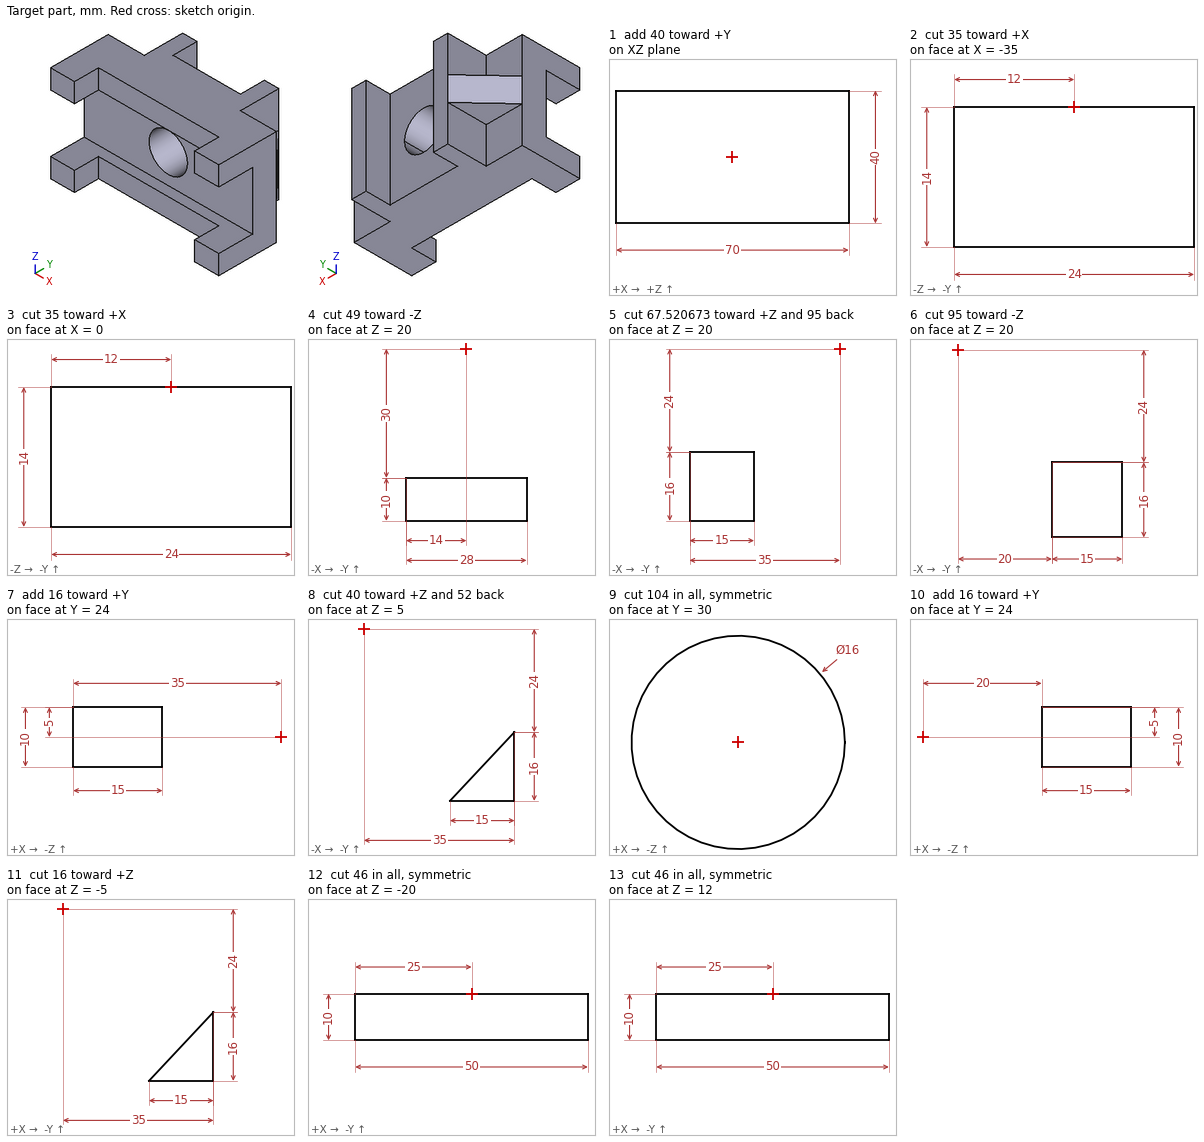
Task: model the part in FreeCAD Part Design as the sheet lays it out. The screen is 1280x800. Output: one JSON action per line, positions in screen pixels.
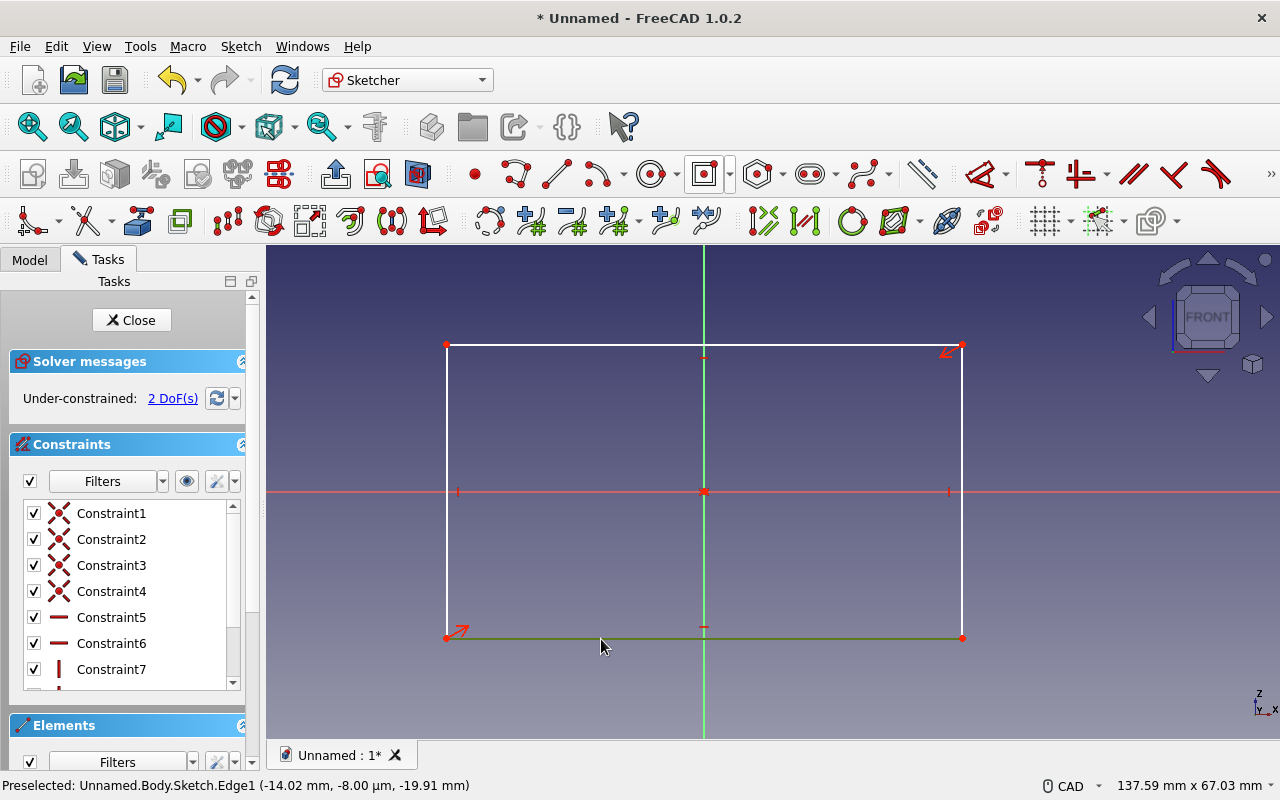
{"action": "key", "text": "l"}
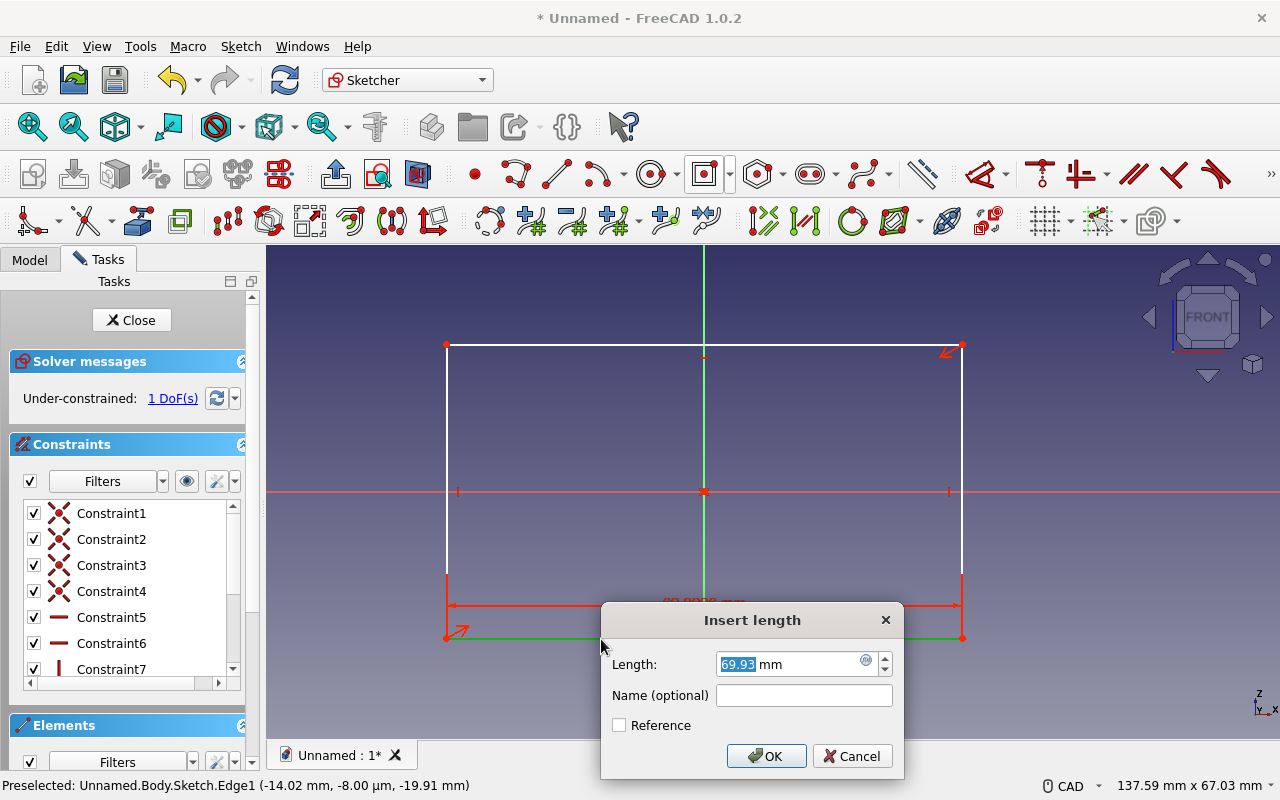
{"action": "type", "text": "70"}
{"action": "key", "text": "Return"}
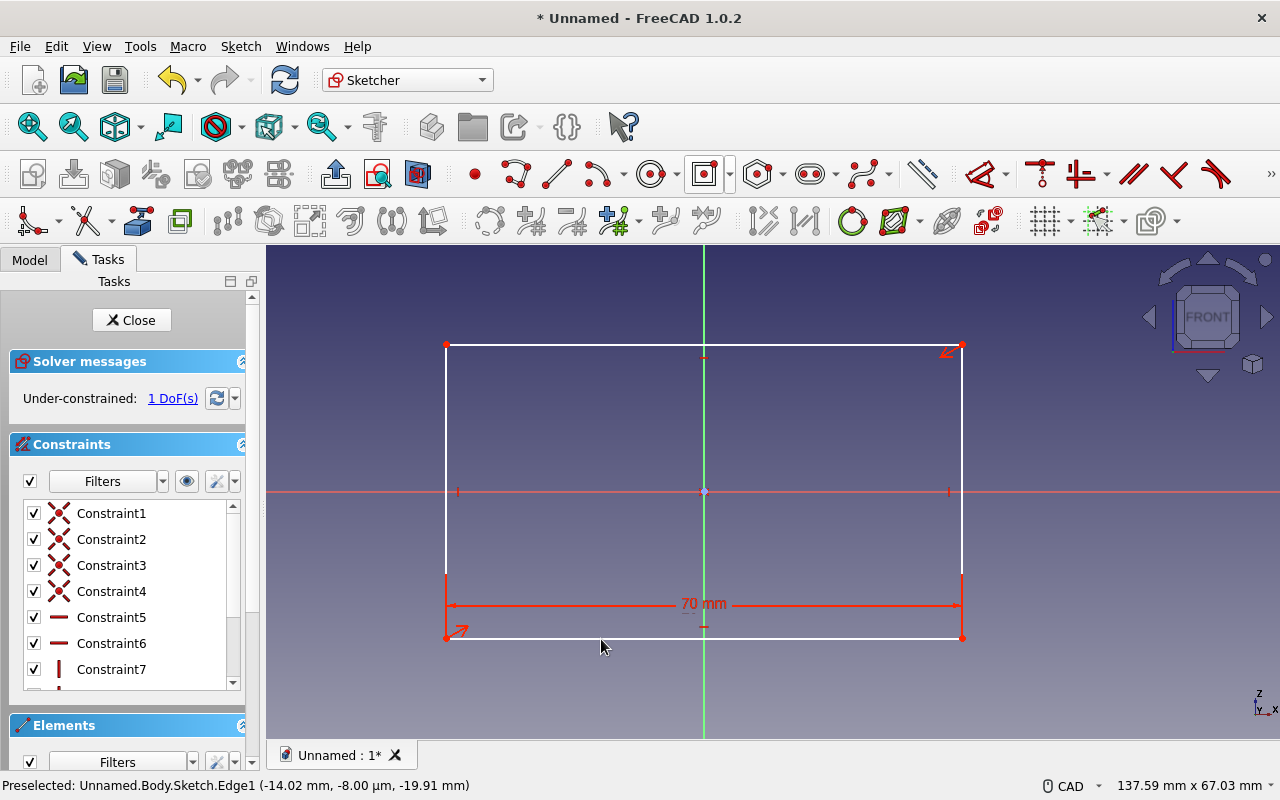
{"action": "left_click", "coordinate": [962, 550]}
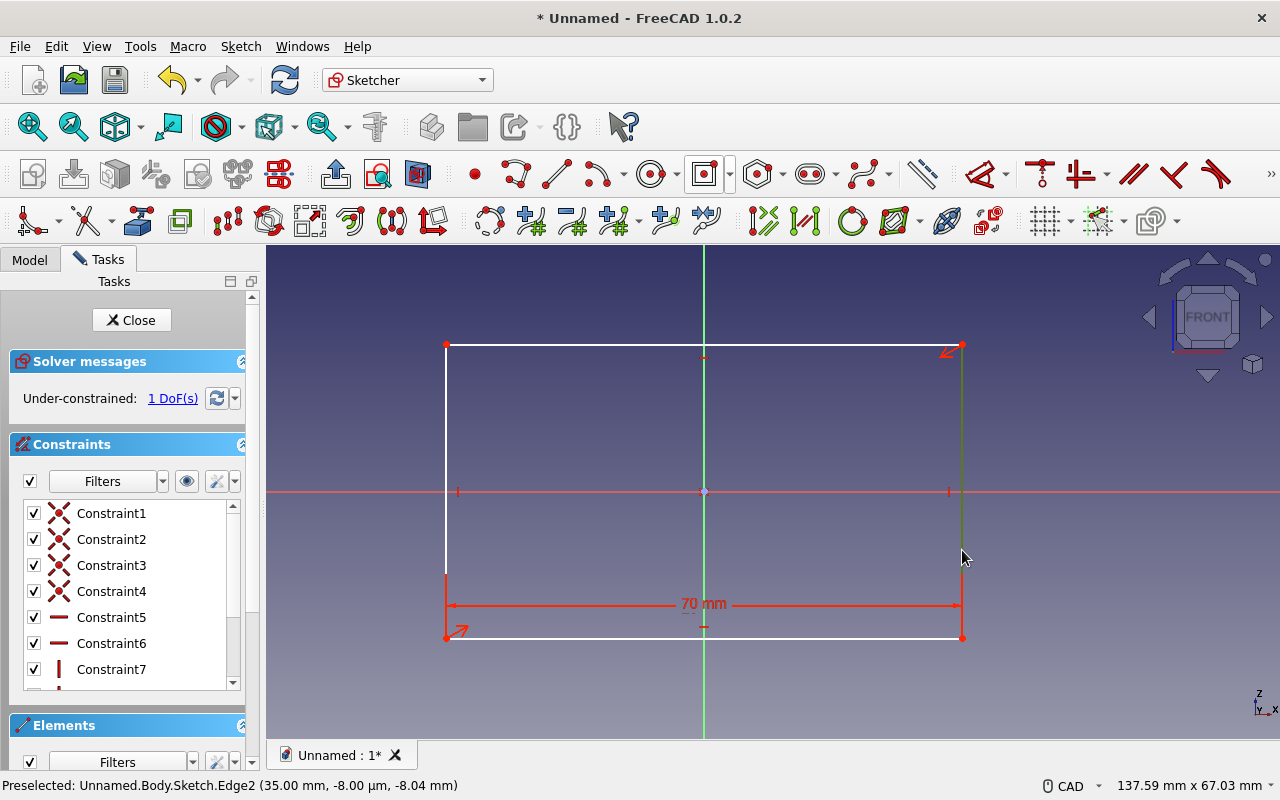
{"action": "key", "text": "i"}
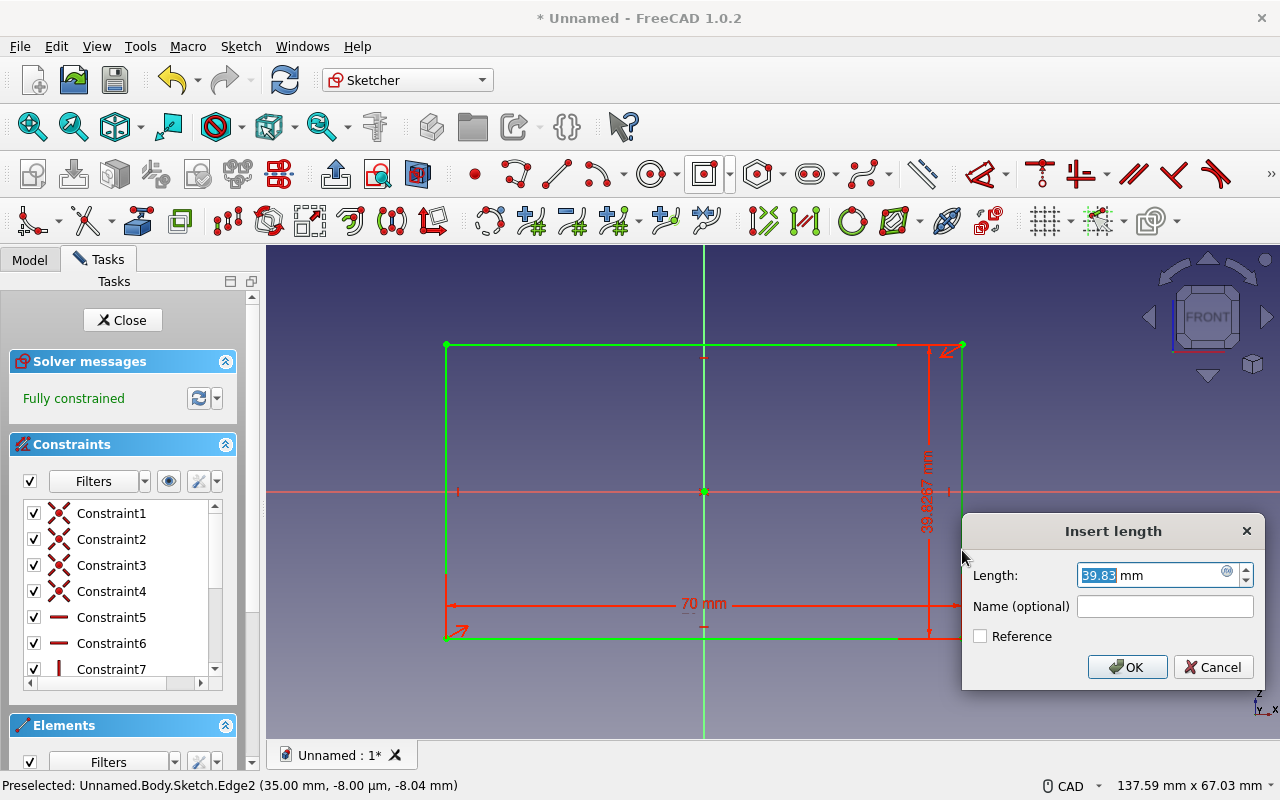
{"action": "type", "text": "40"}
{"action": "key", "text": "Return"}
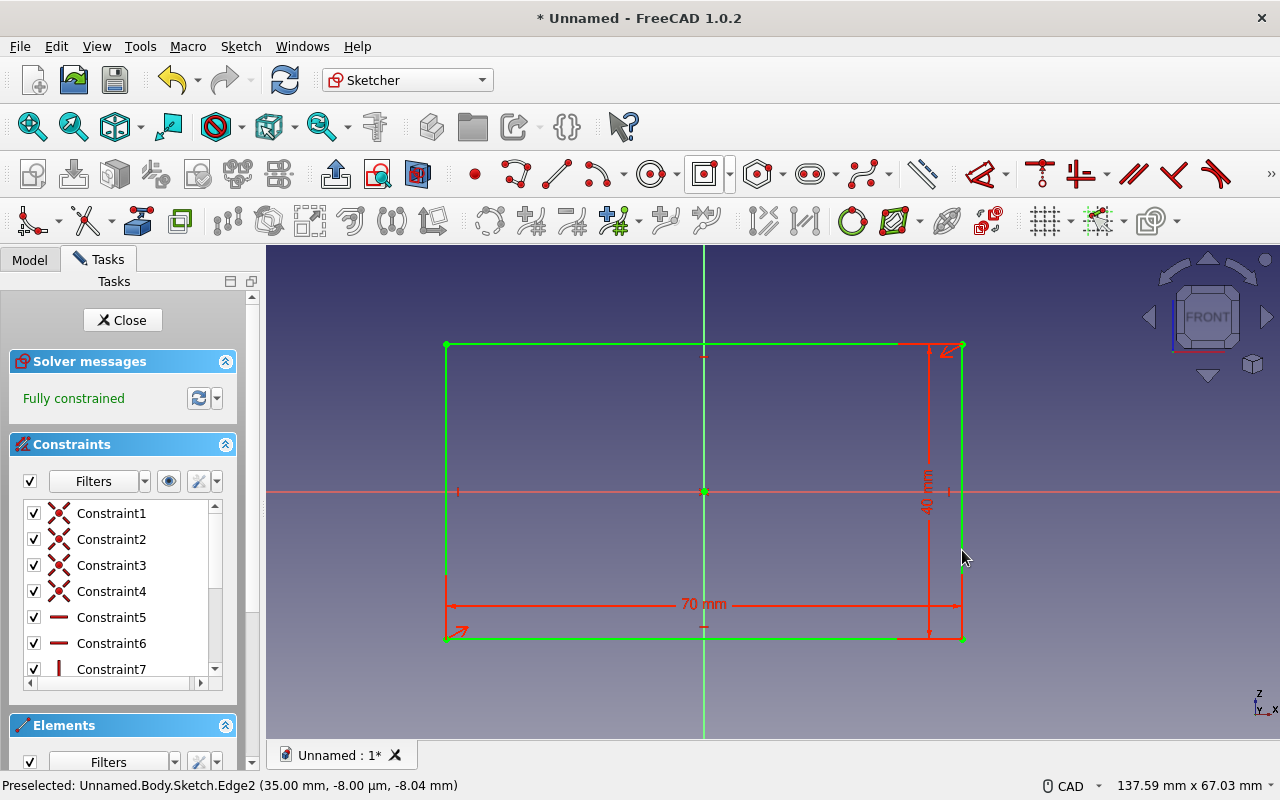
{"action": "left_click", "coordinate": [123, 320]}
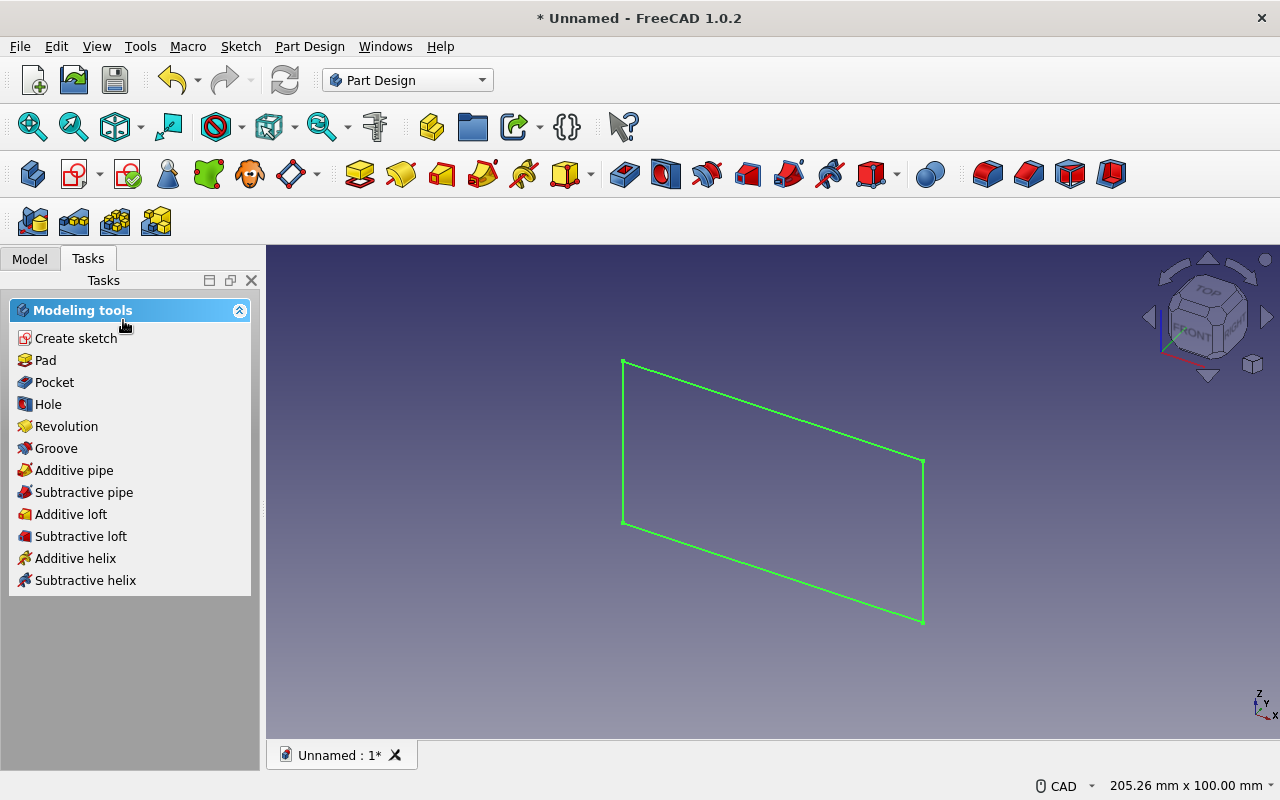
{"action": "left_click", "coordinate": [360, 174]}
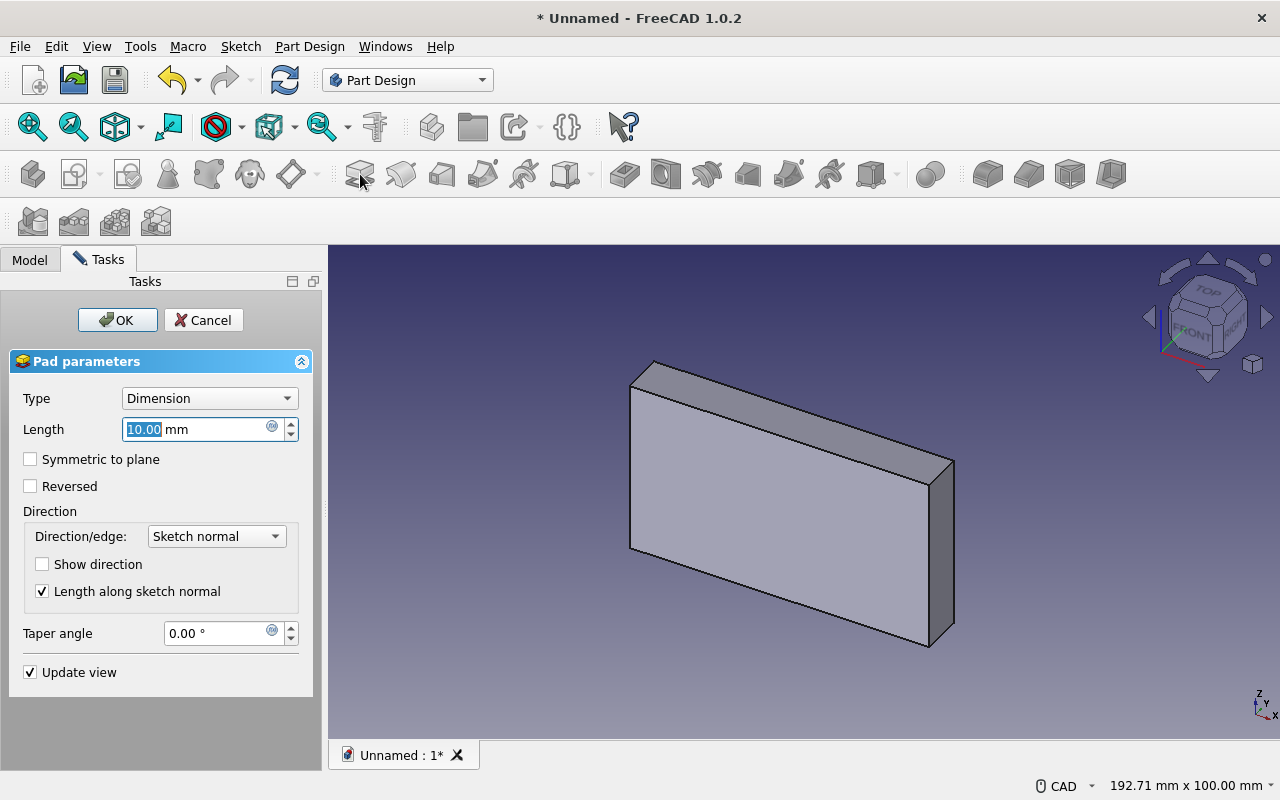
{"action": "type", "text": "40"}
{"action": "key", "text": "Tab"}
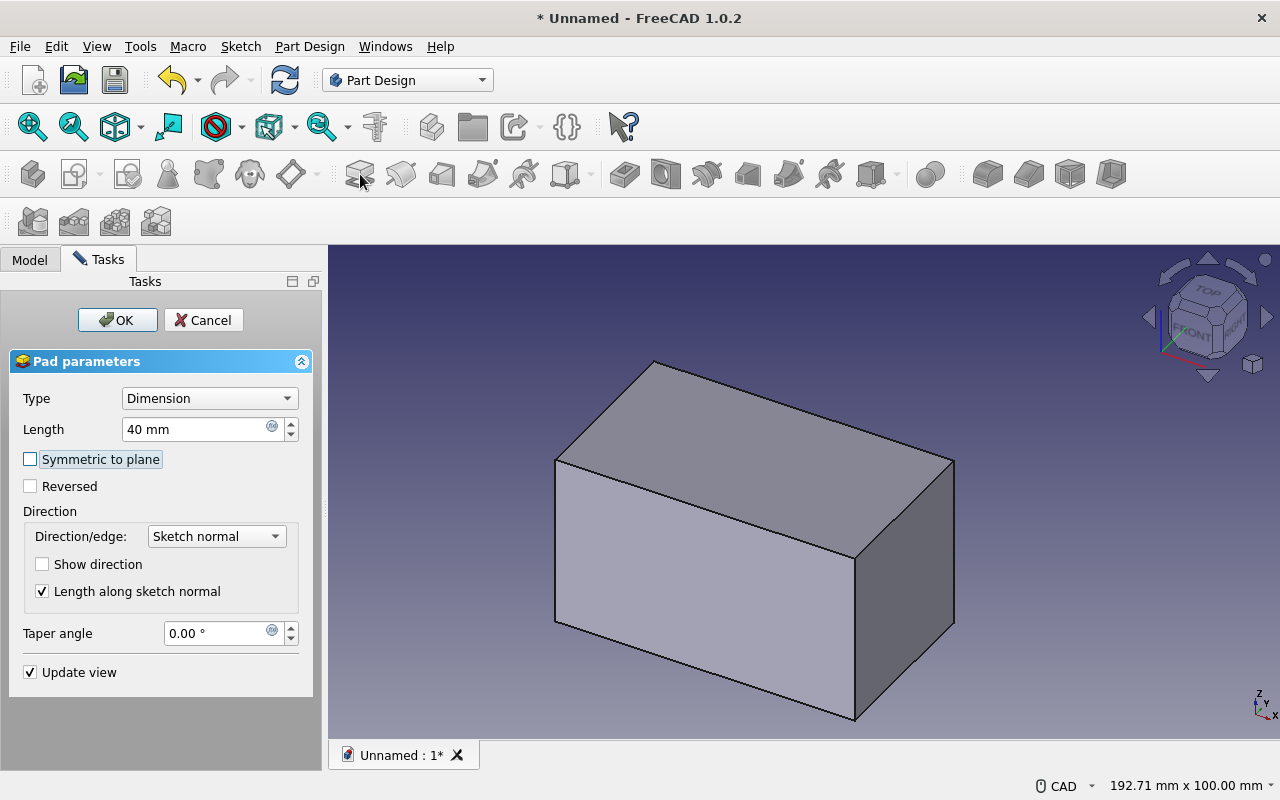
{"action": "left_click", "coordinate": [31, 486]}